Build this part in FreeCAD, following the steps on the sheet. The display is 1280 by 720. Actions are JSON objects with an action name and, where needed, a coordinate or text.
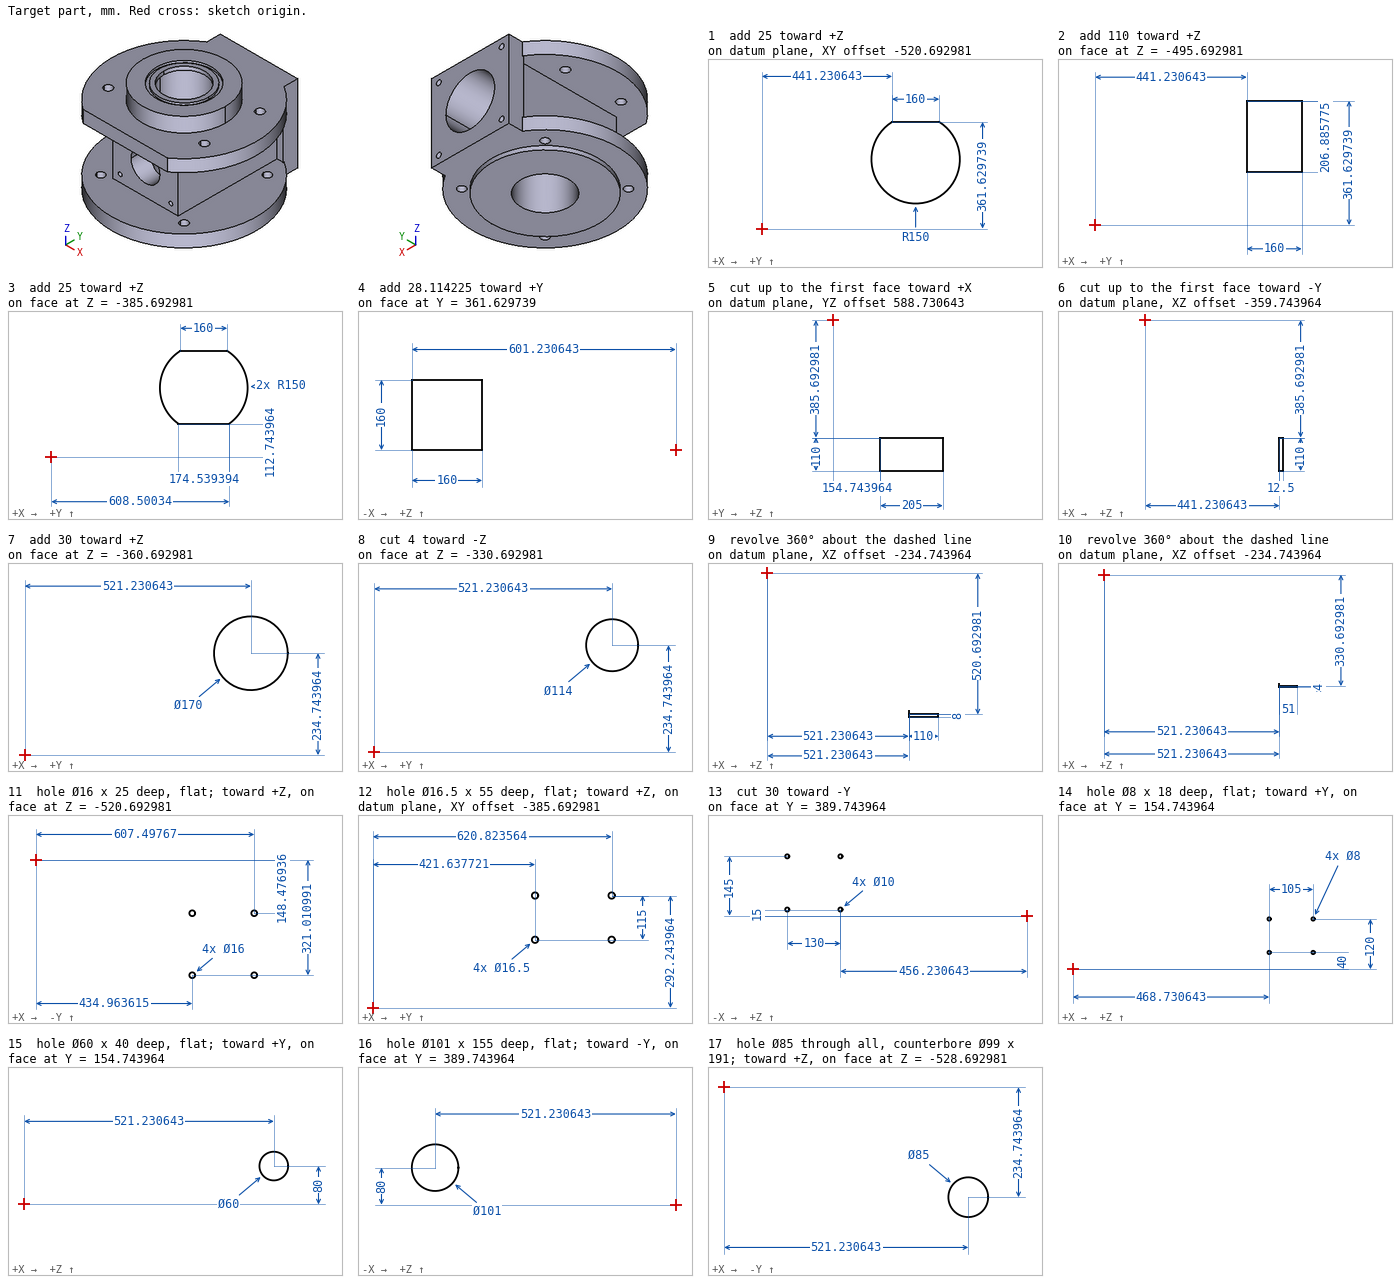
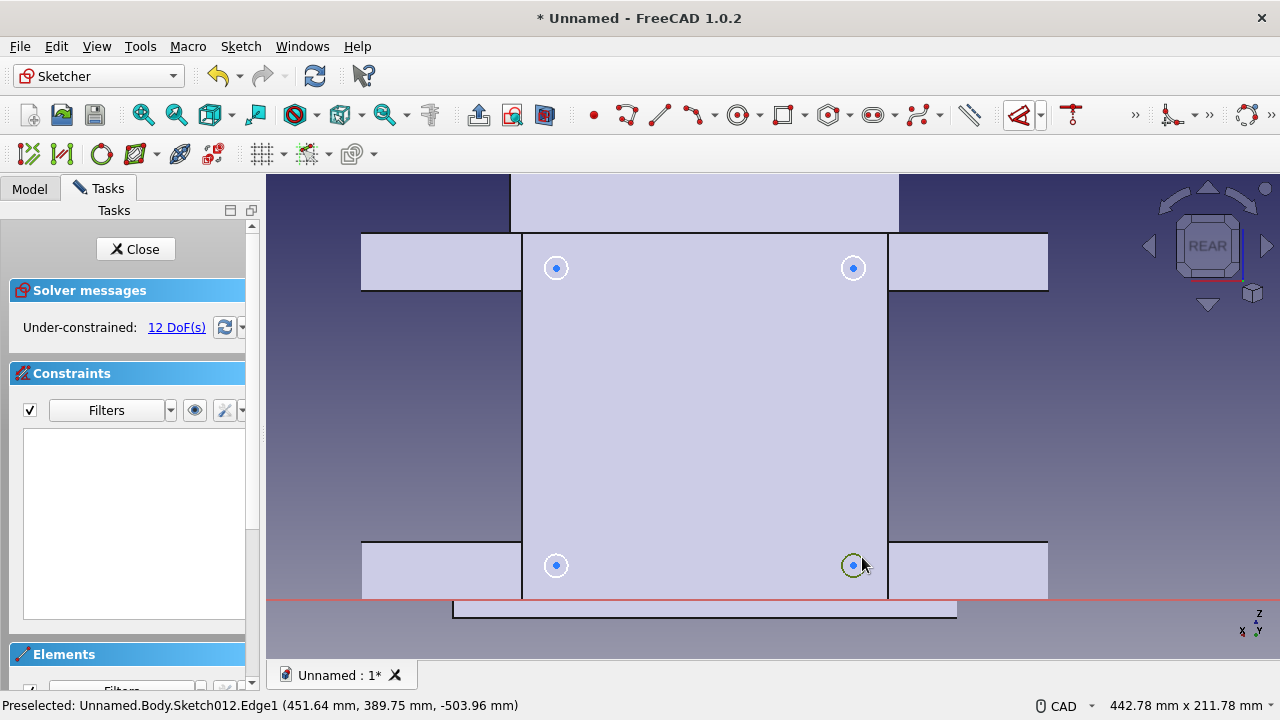
{"action": "left_click", "coordinate": [564, 558]}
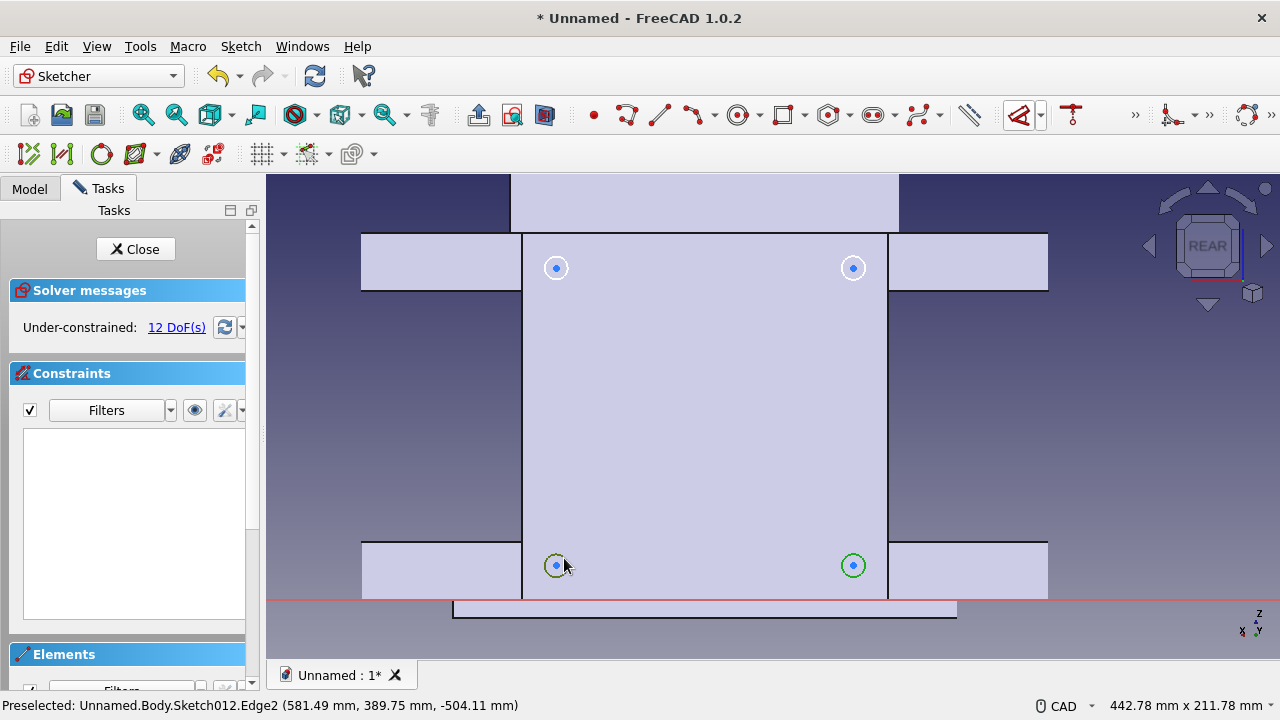
{"action": "left_click", "coordinate": [564, 260]}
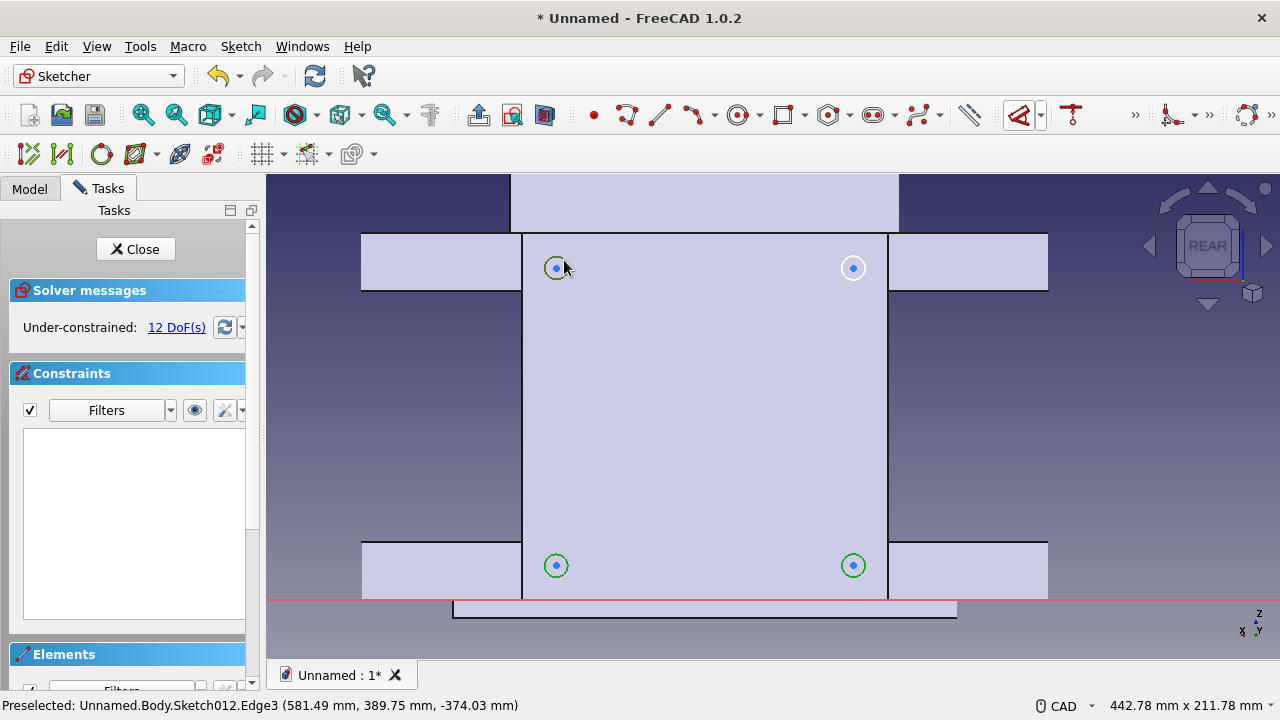
{"action": "left_click", "coordinate": [862, 260]}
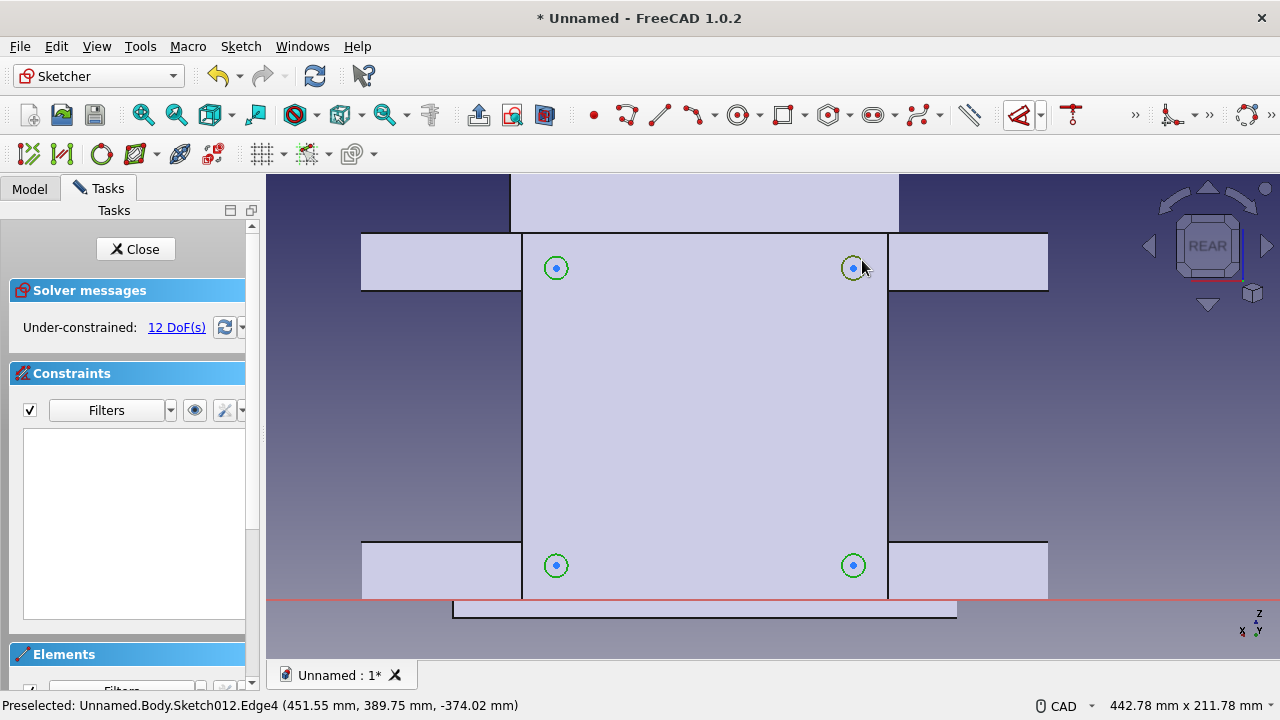
{"action": "key", "text": "e"}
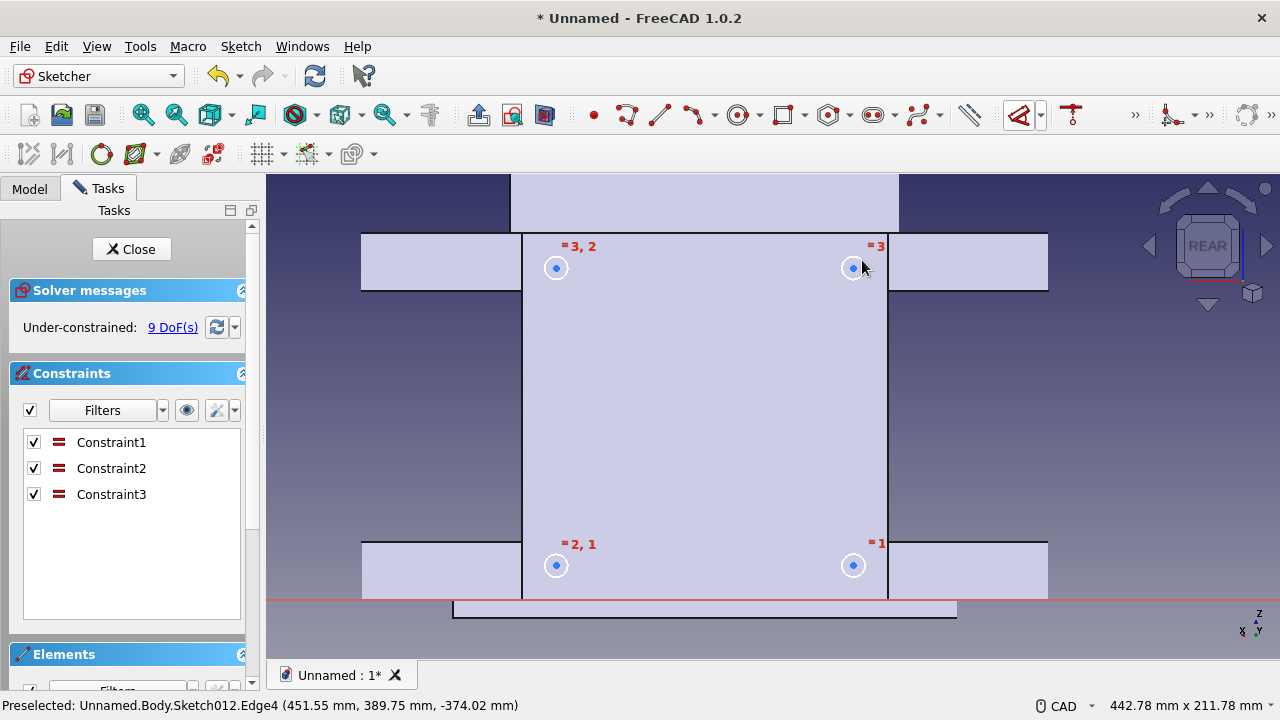
{"action": "left_click", "coordinate": [854, 566]}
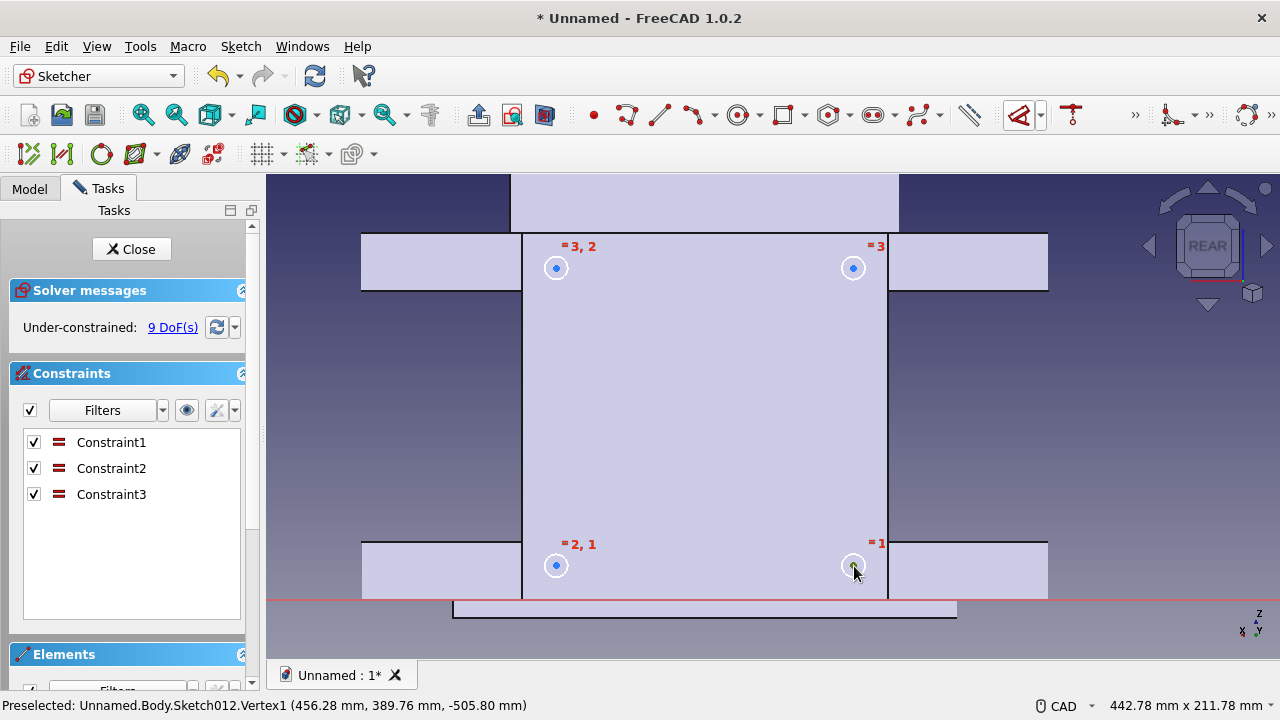
{"action": "left_click", "coordinate": [556, 566]}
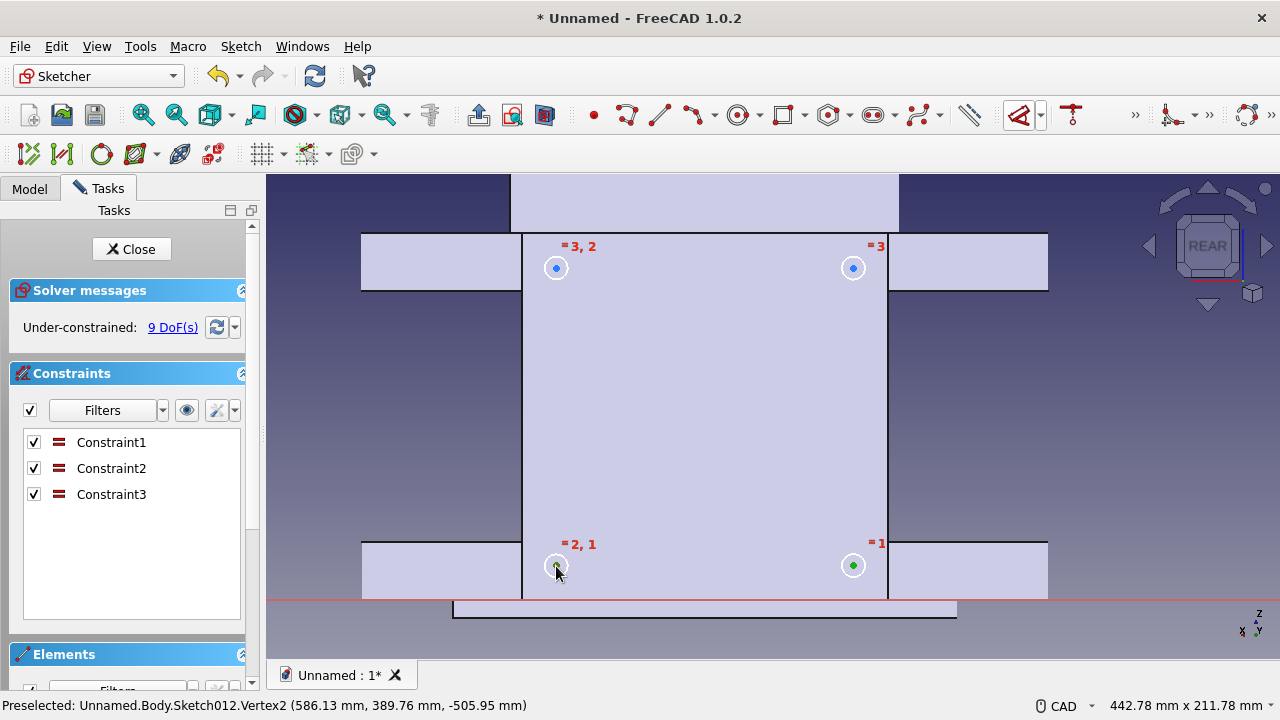
{"action": "key", "text": "h"}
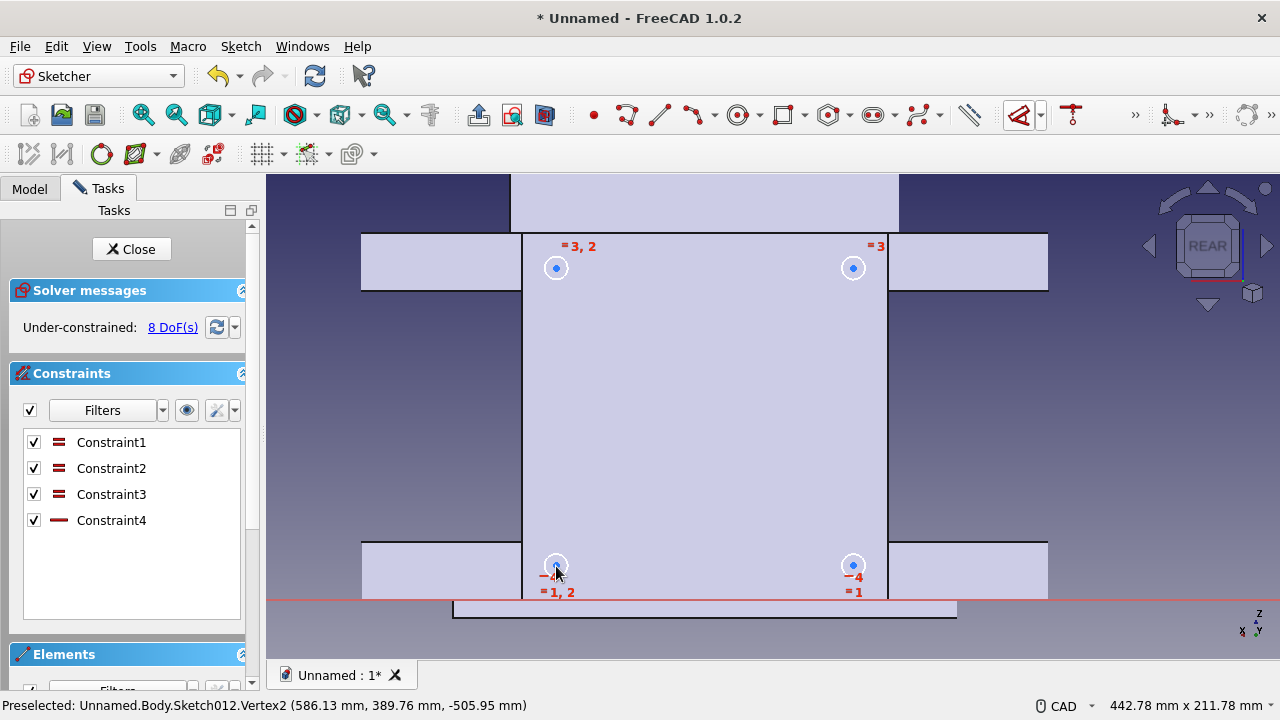
{"action": "left_click", "coordinate": [556, 566]}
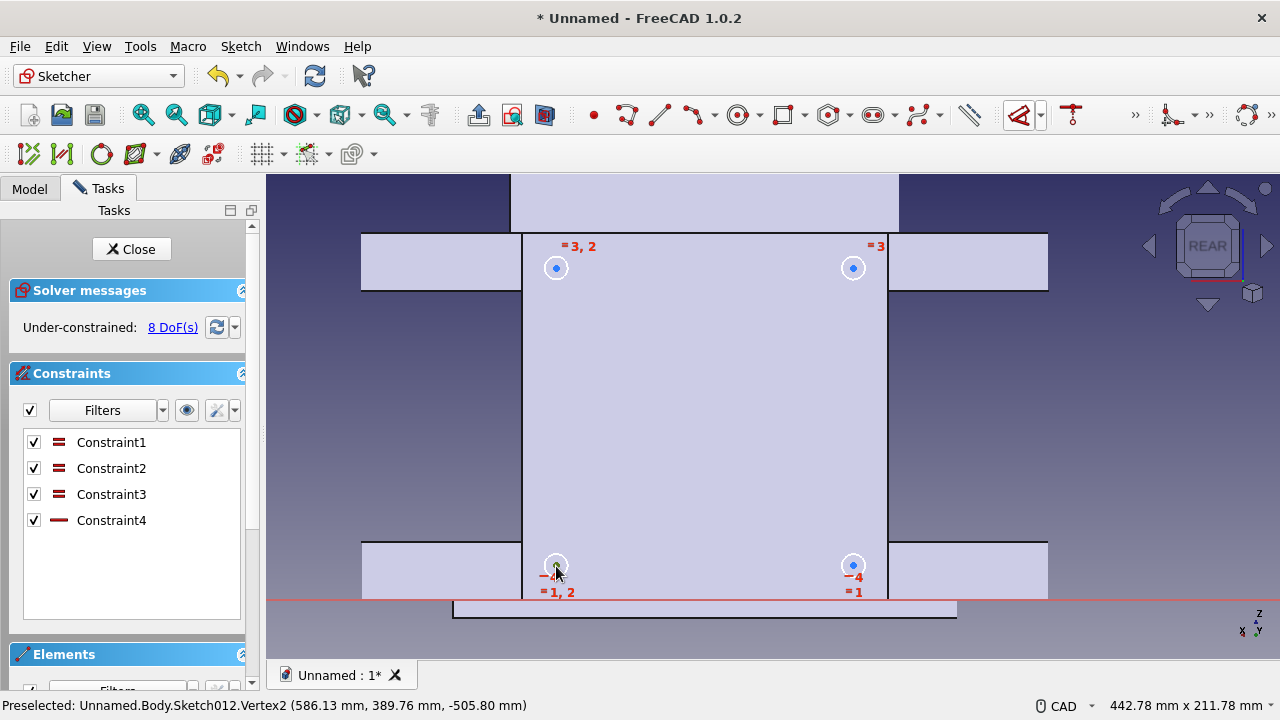
{"action": "left_click", "coordinate": [556, 268]}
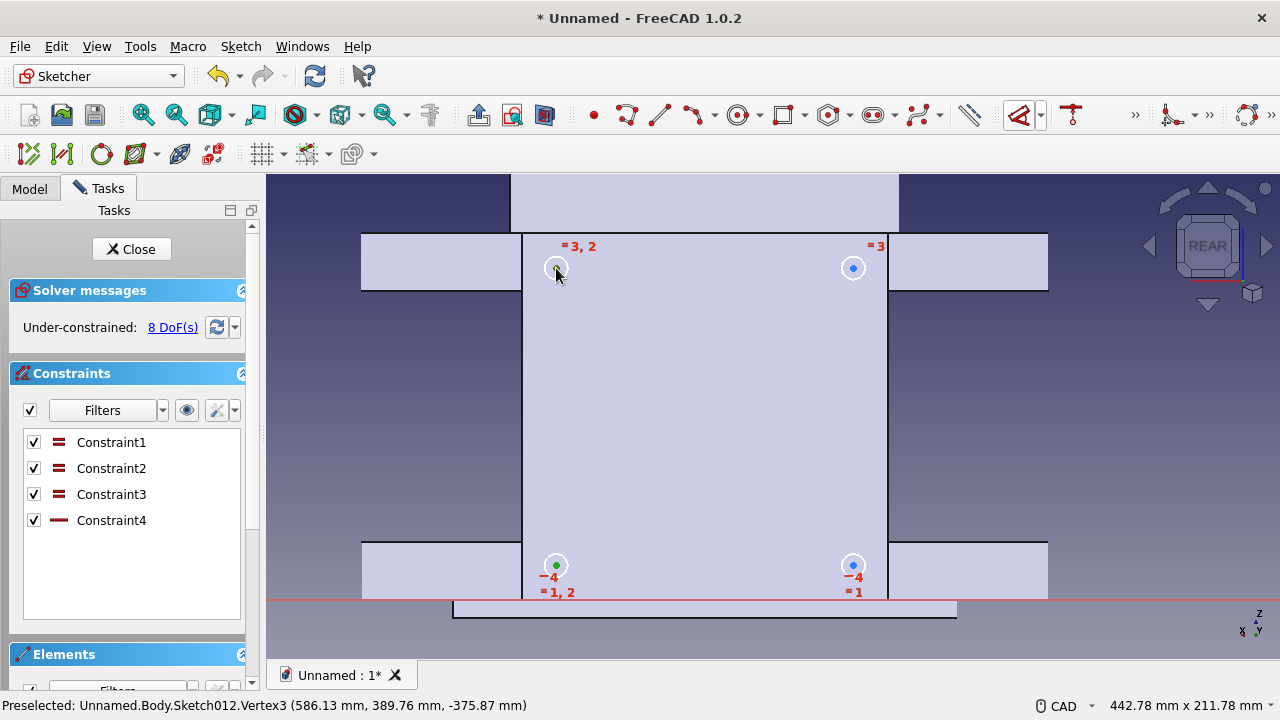
{"action": "key", "text": "v"}